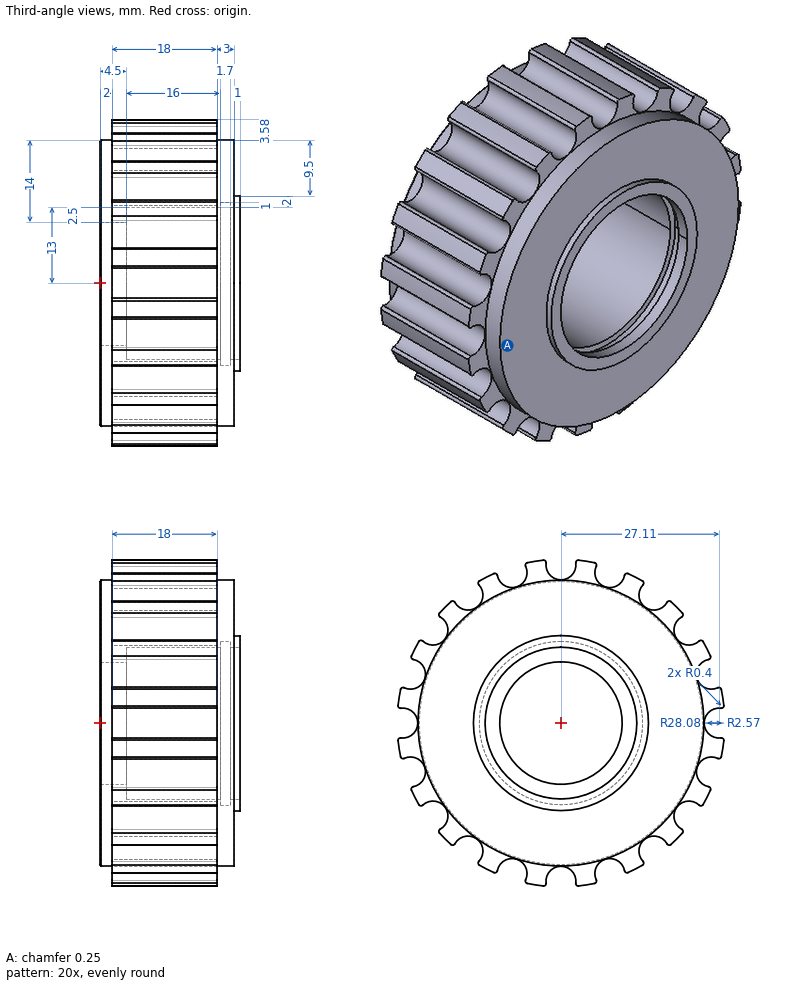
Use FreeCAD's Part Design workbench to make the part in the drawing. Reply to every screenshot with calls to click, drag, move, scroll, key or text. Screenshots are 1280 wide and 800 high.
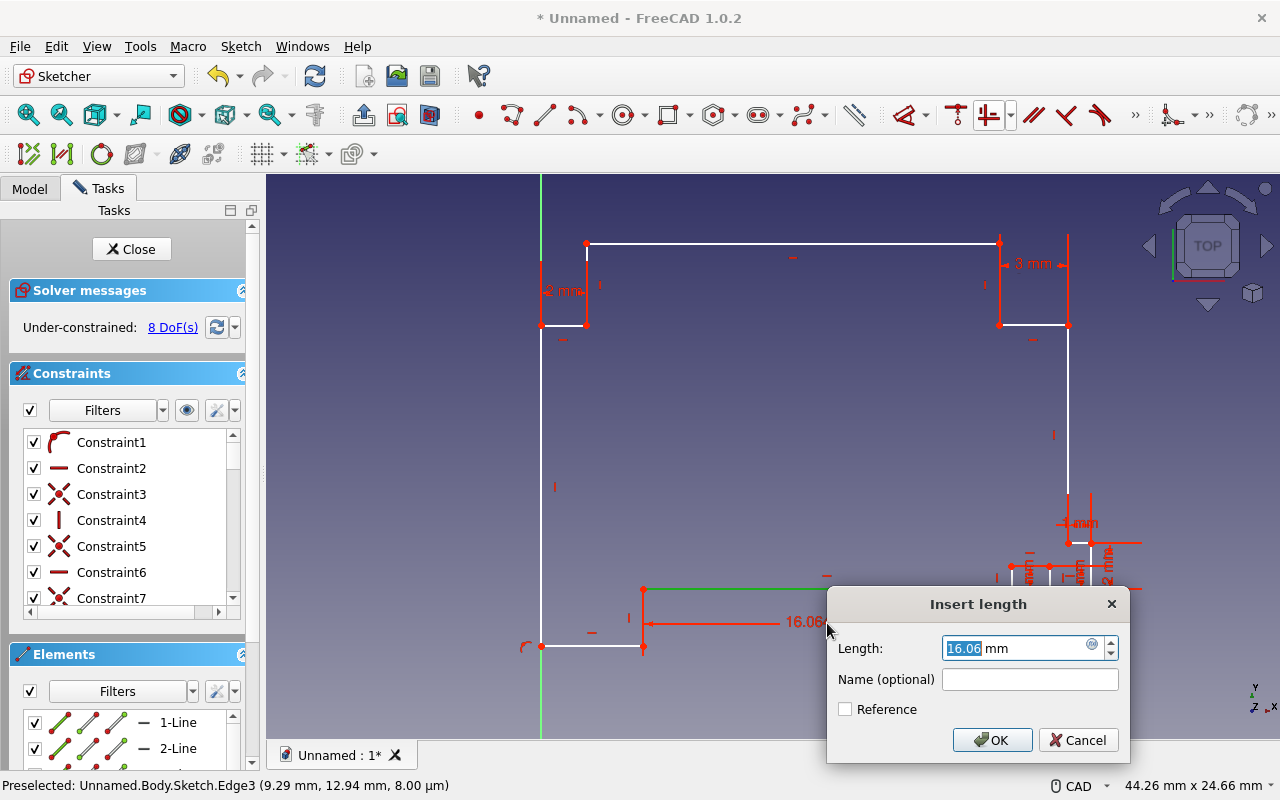
text(16)
key(Return)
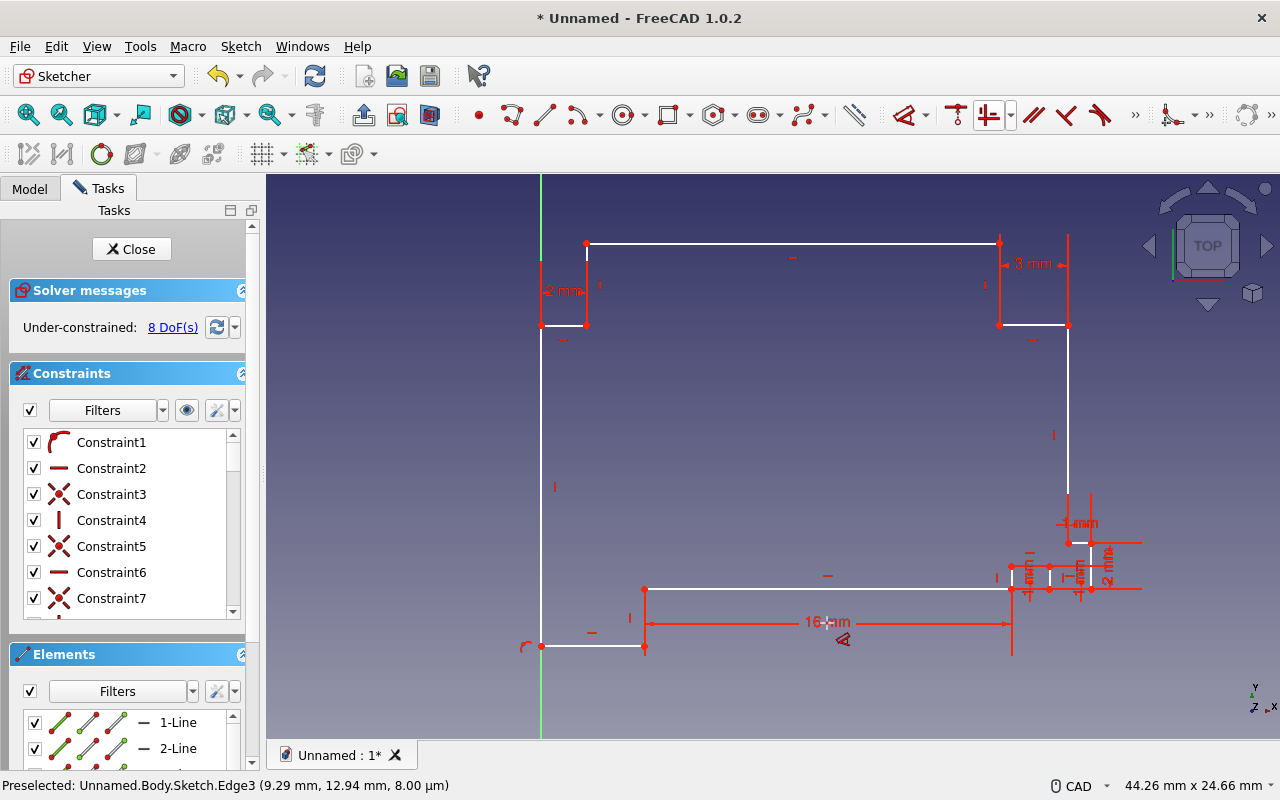
click(876, 244)
click(793, 210)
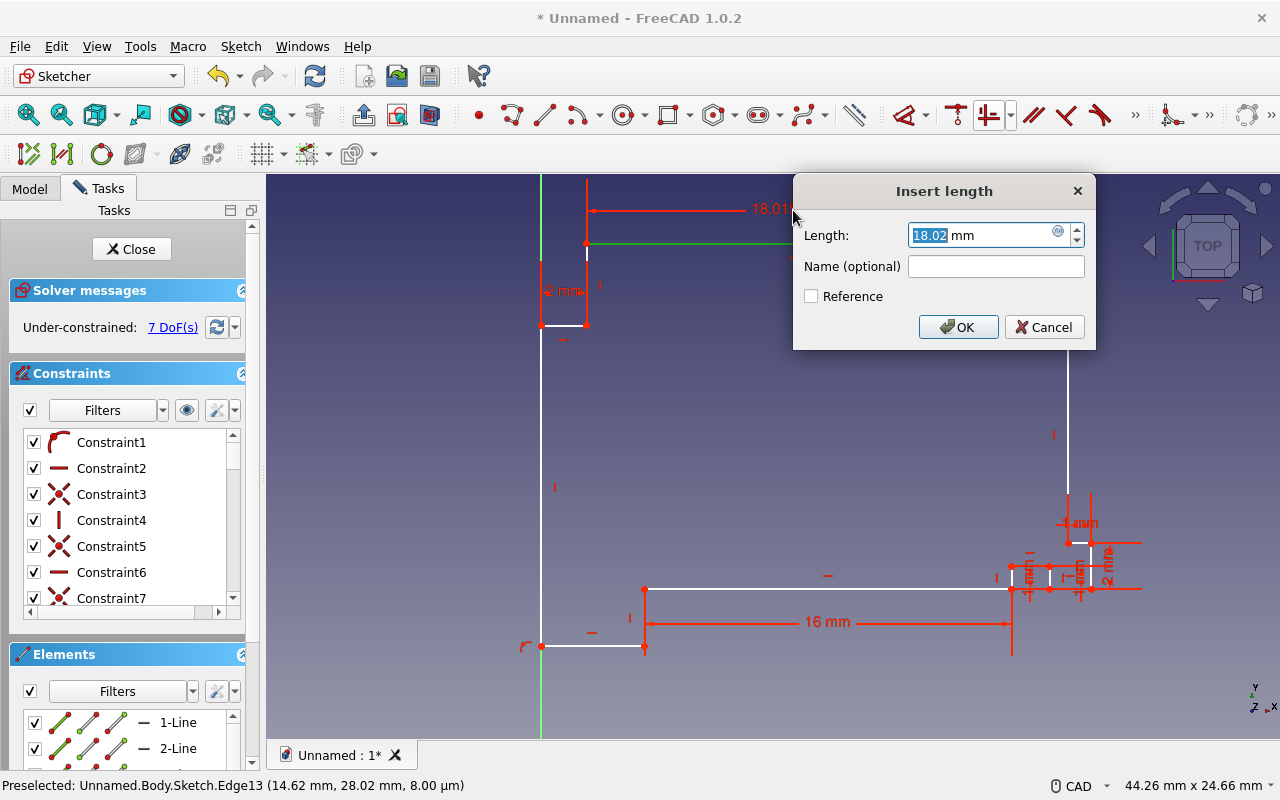
text(18)
key(Return)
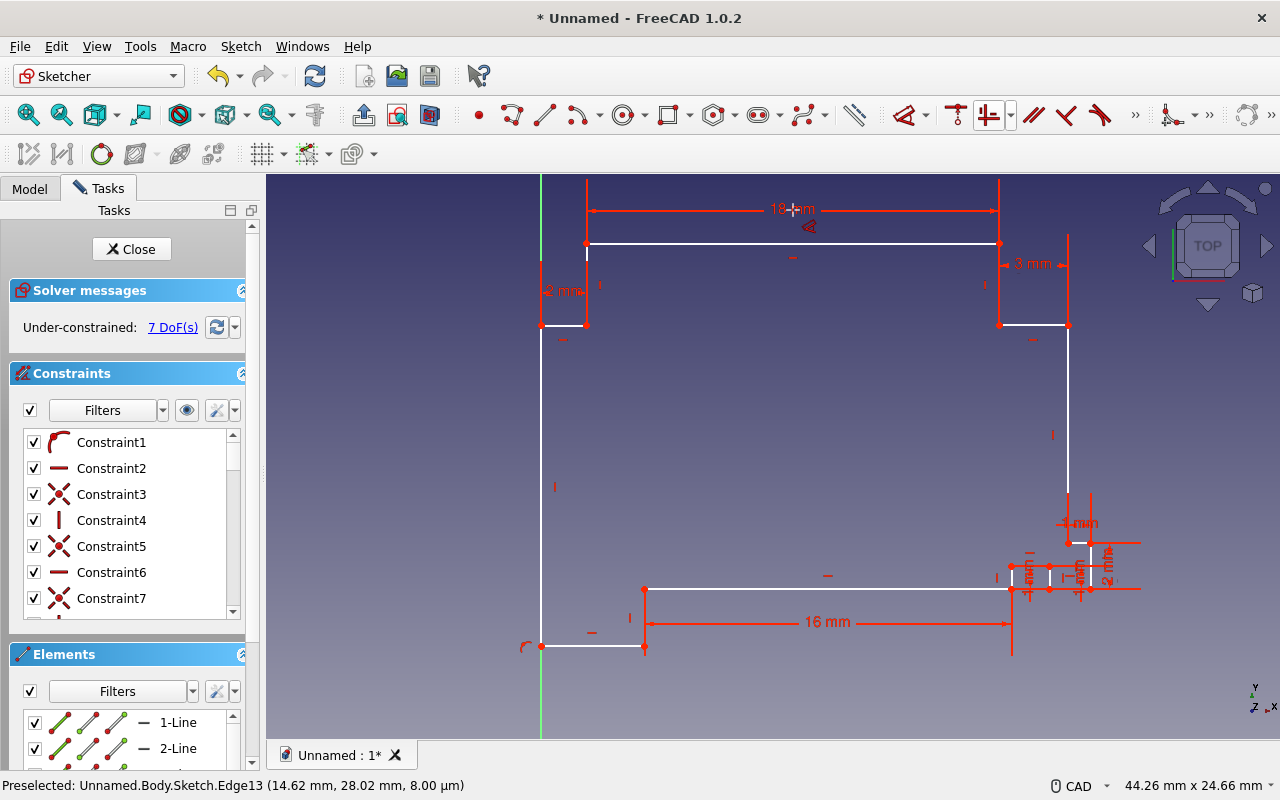
click(541, 422)
click(507, 486)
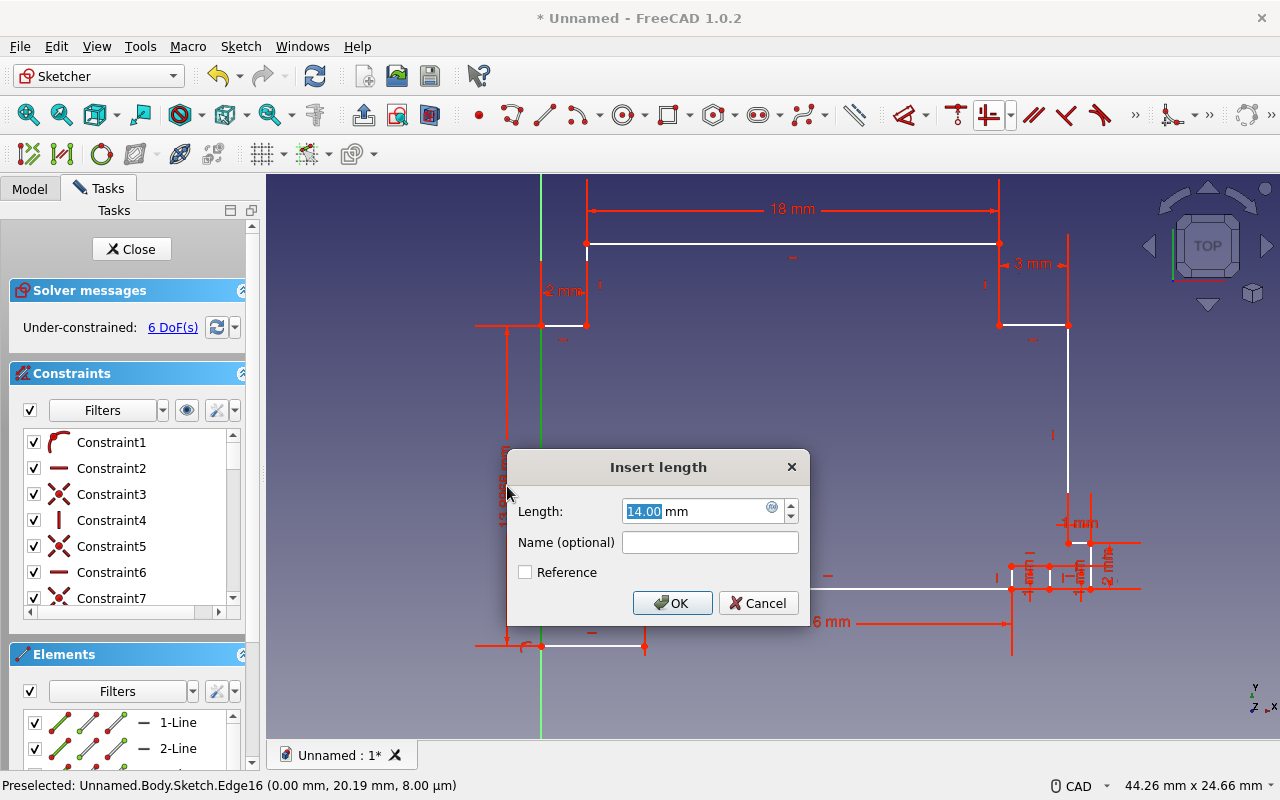
text(14)
key(Return)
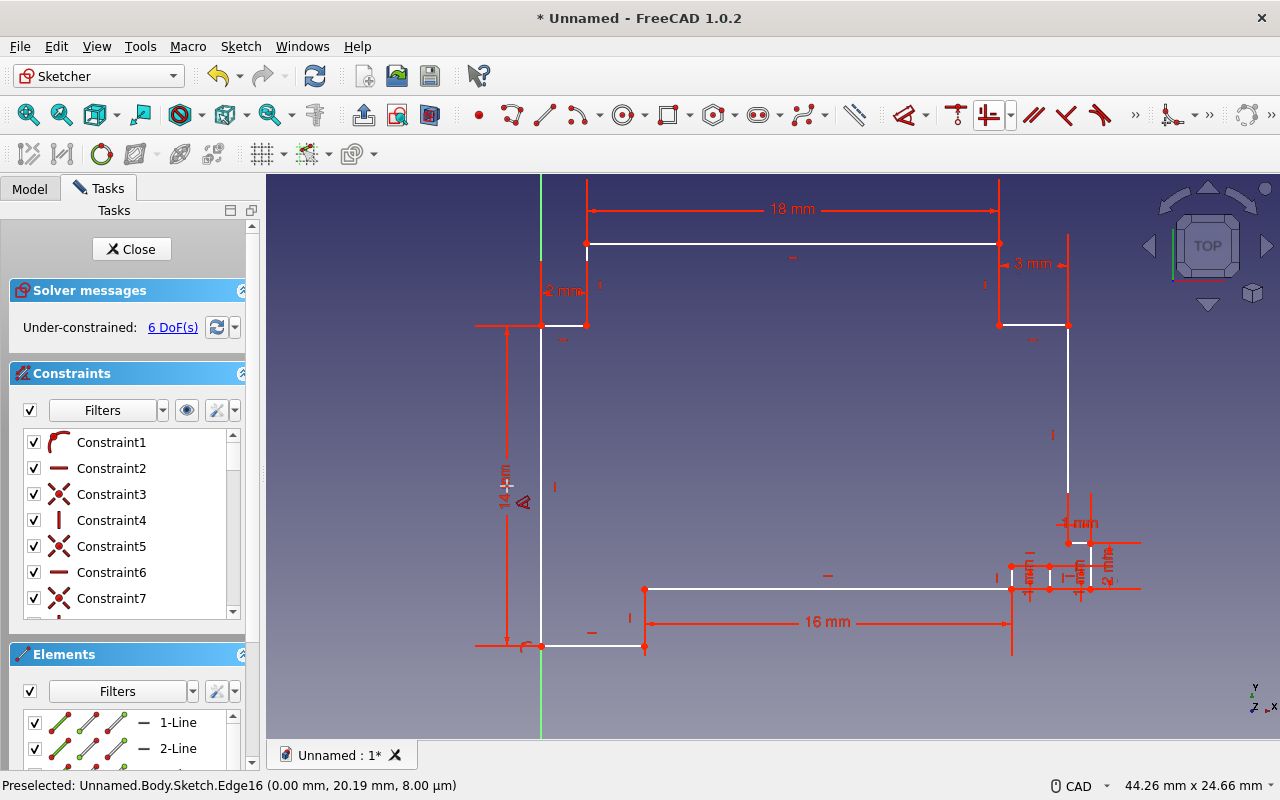
click(572, 646)
click(593, 680)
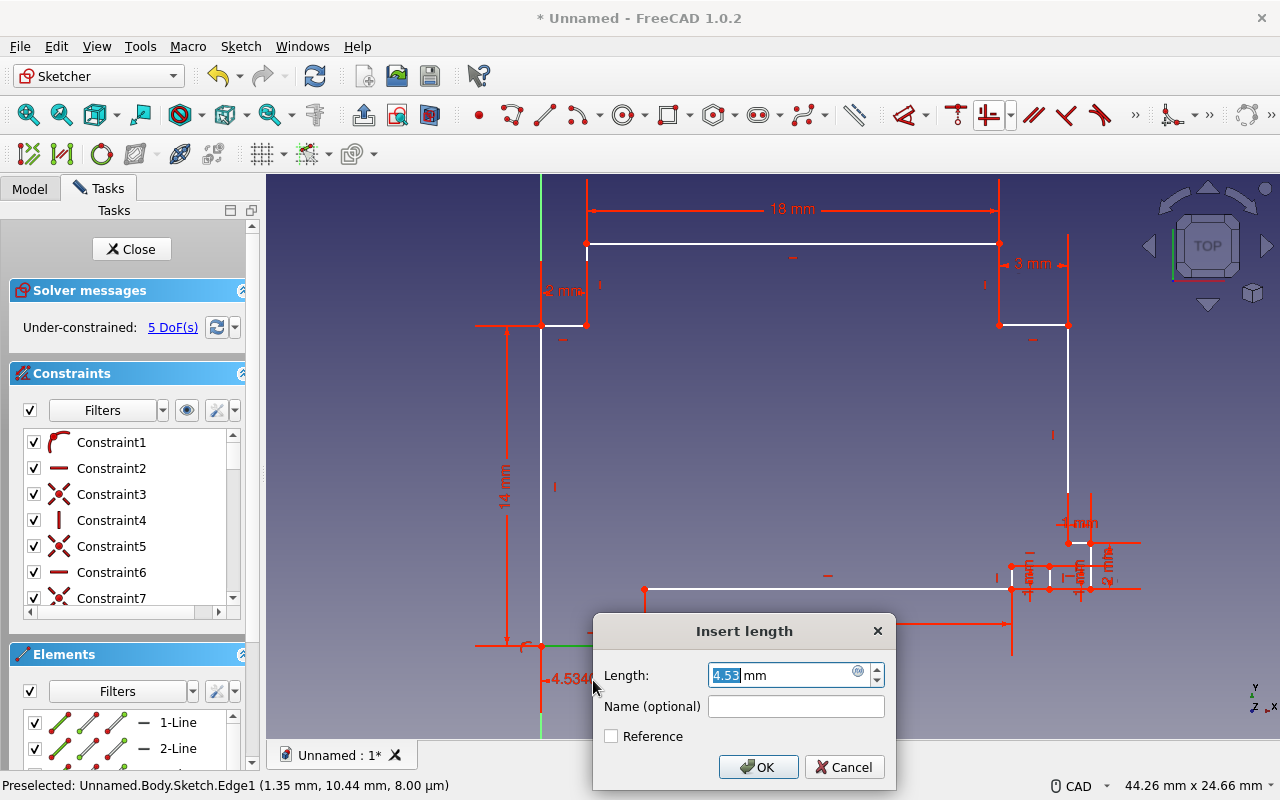
text(4.5)
key(Return)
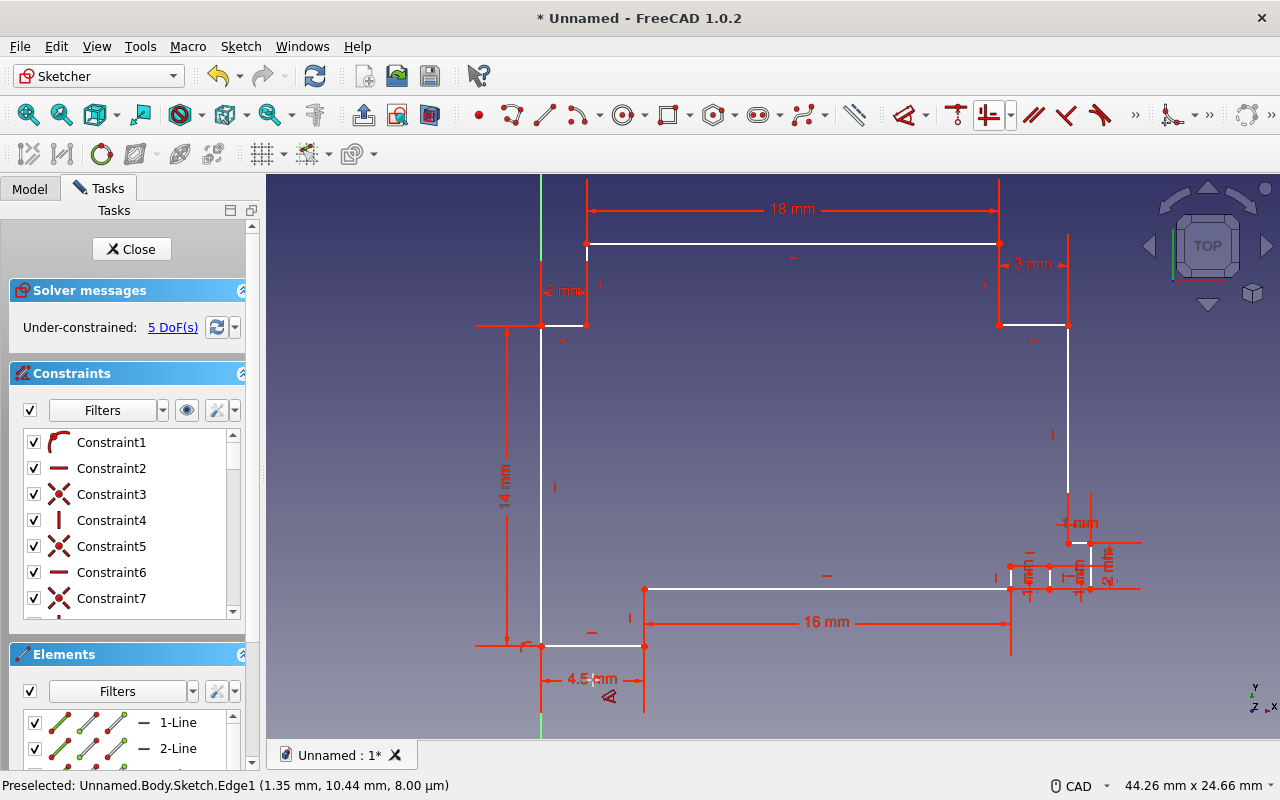
click(644, 629)
click(610, 618)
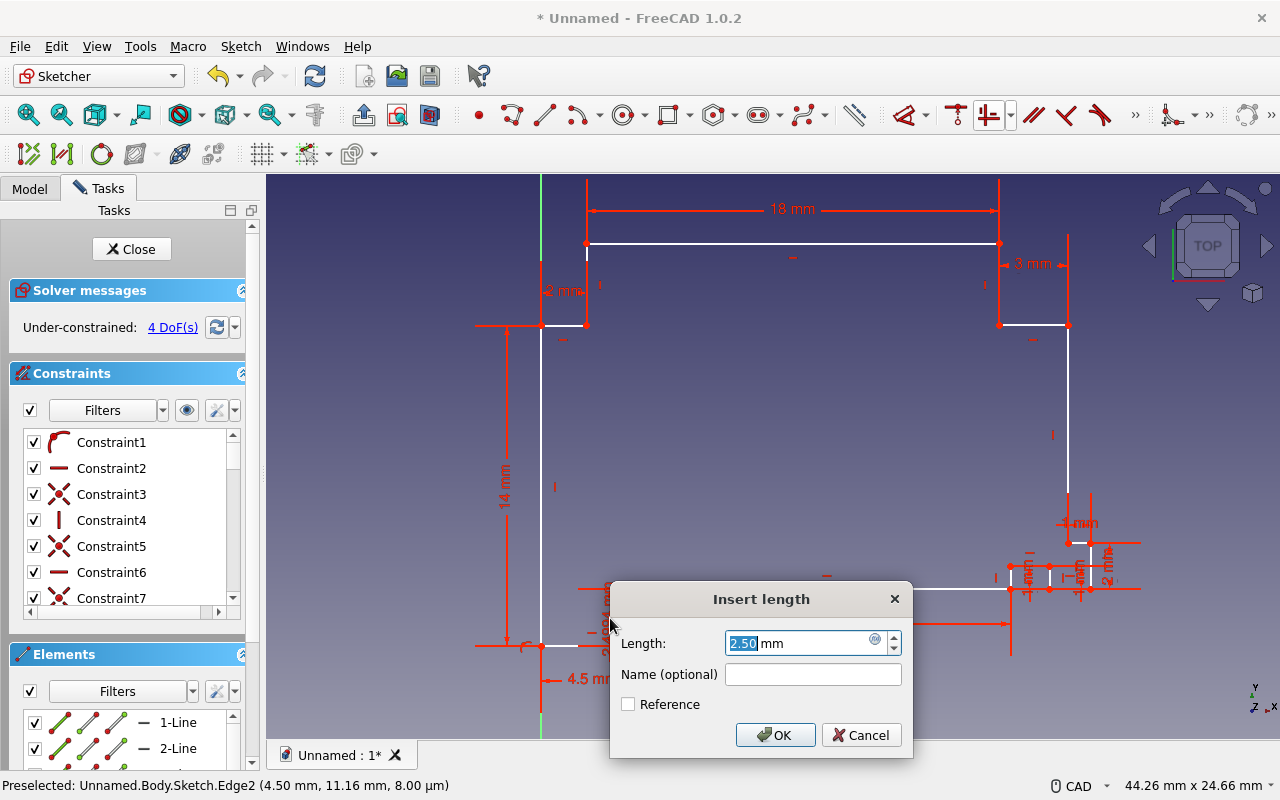
text(2.5)
key(Return)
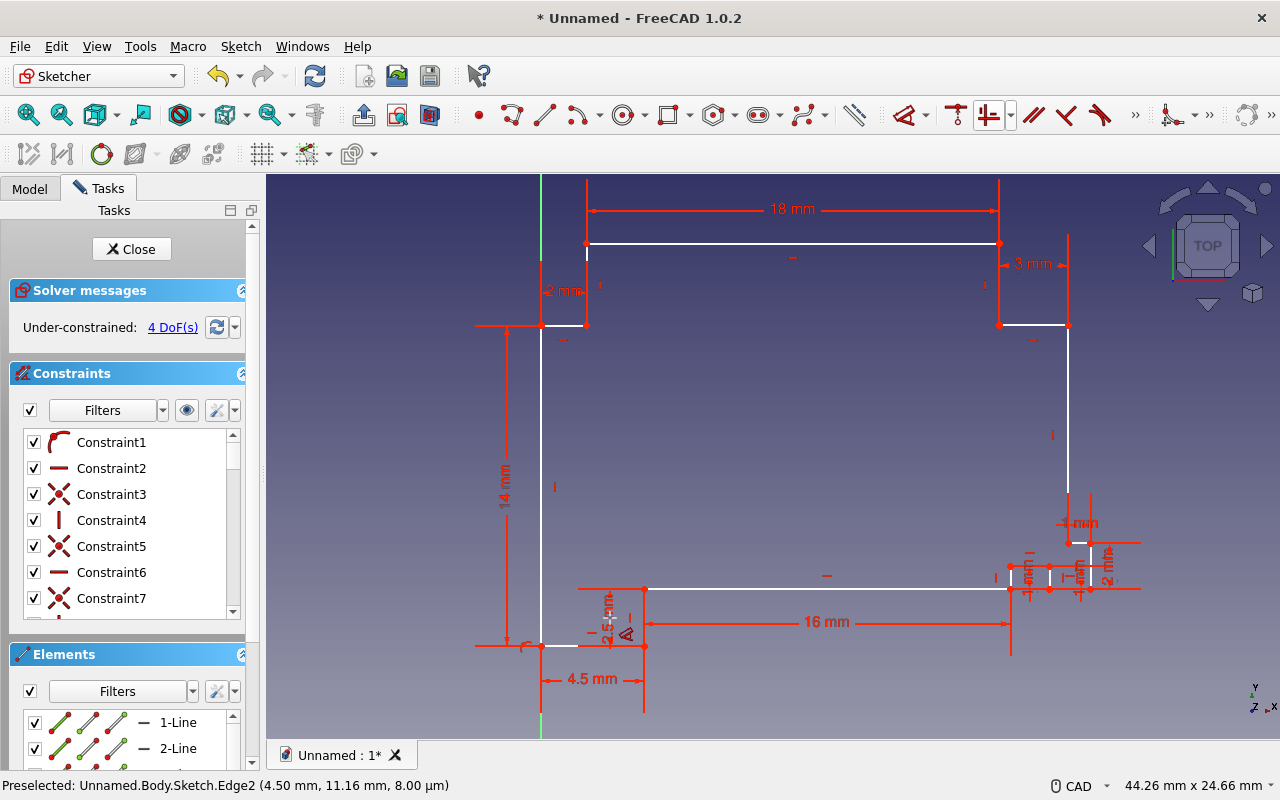
click(1022, 566)
click(1030, 600)